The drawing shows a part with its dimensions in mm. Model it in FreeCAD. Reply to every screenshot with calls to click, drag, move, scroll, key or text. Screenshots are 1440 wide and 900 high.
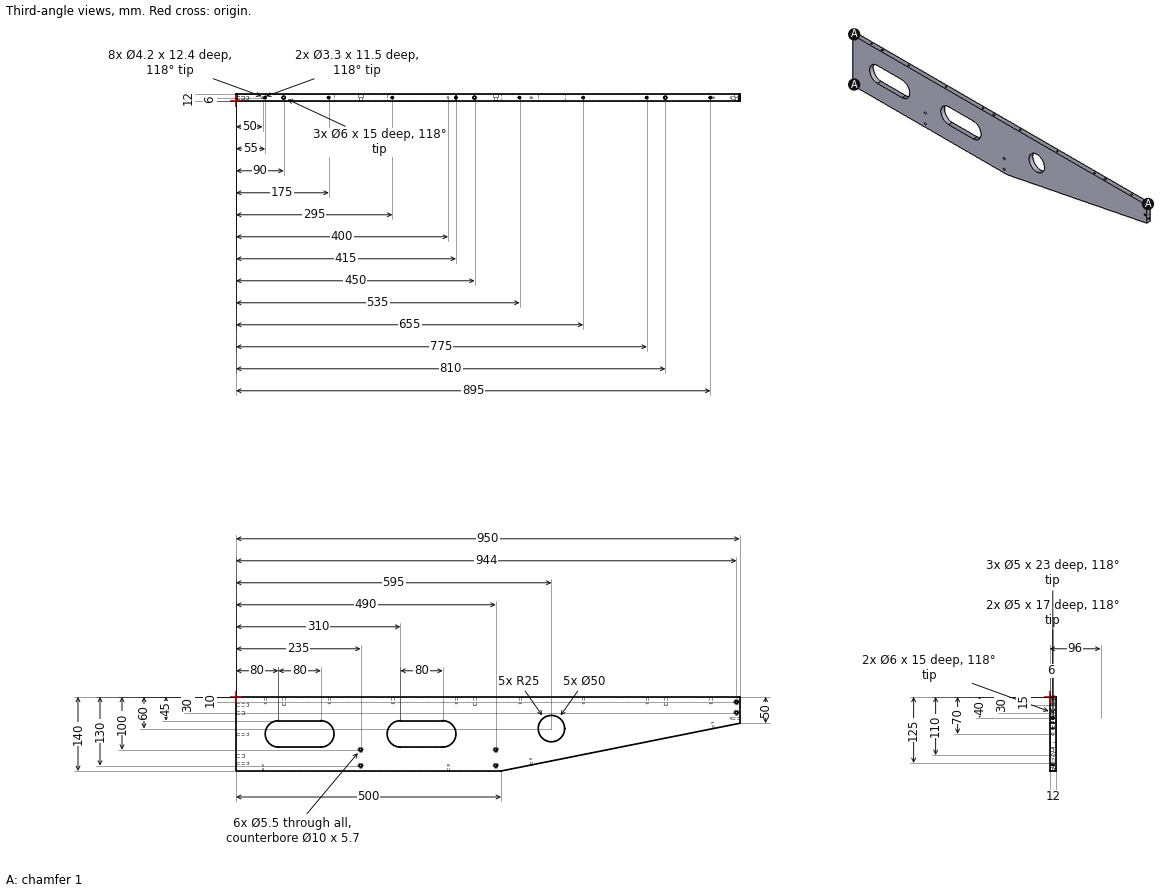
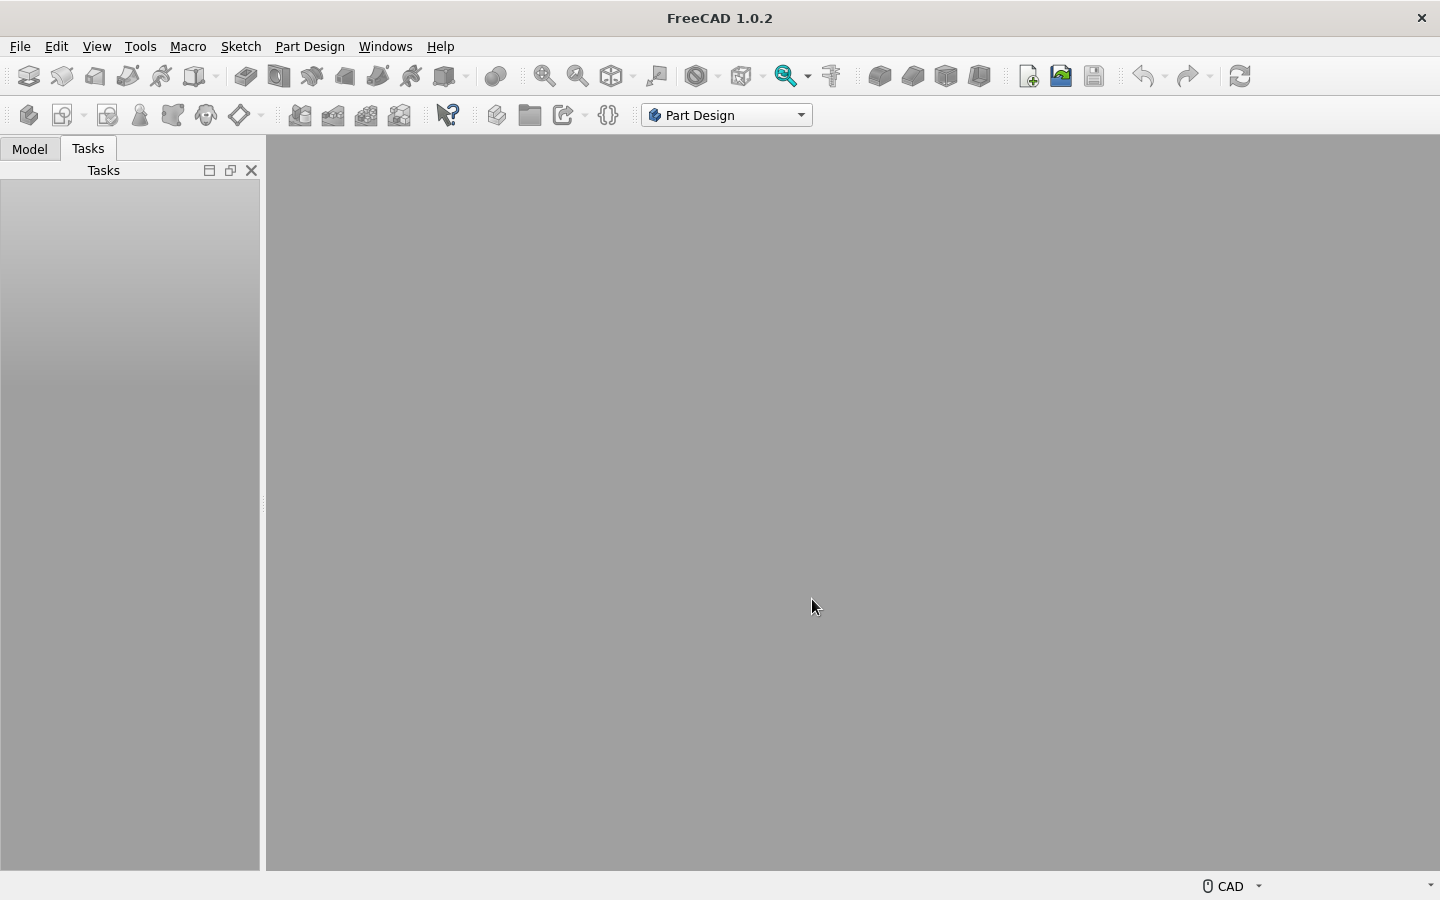
click(1028, 76)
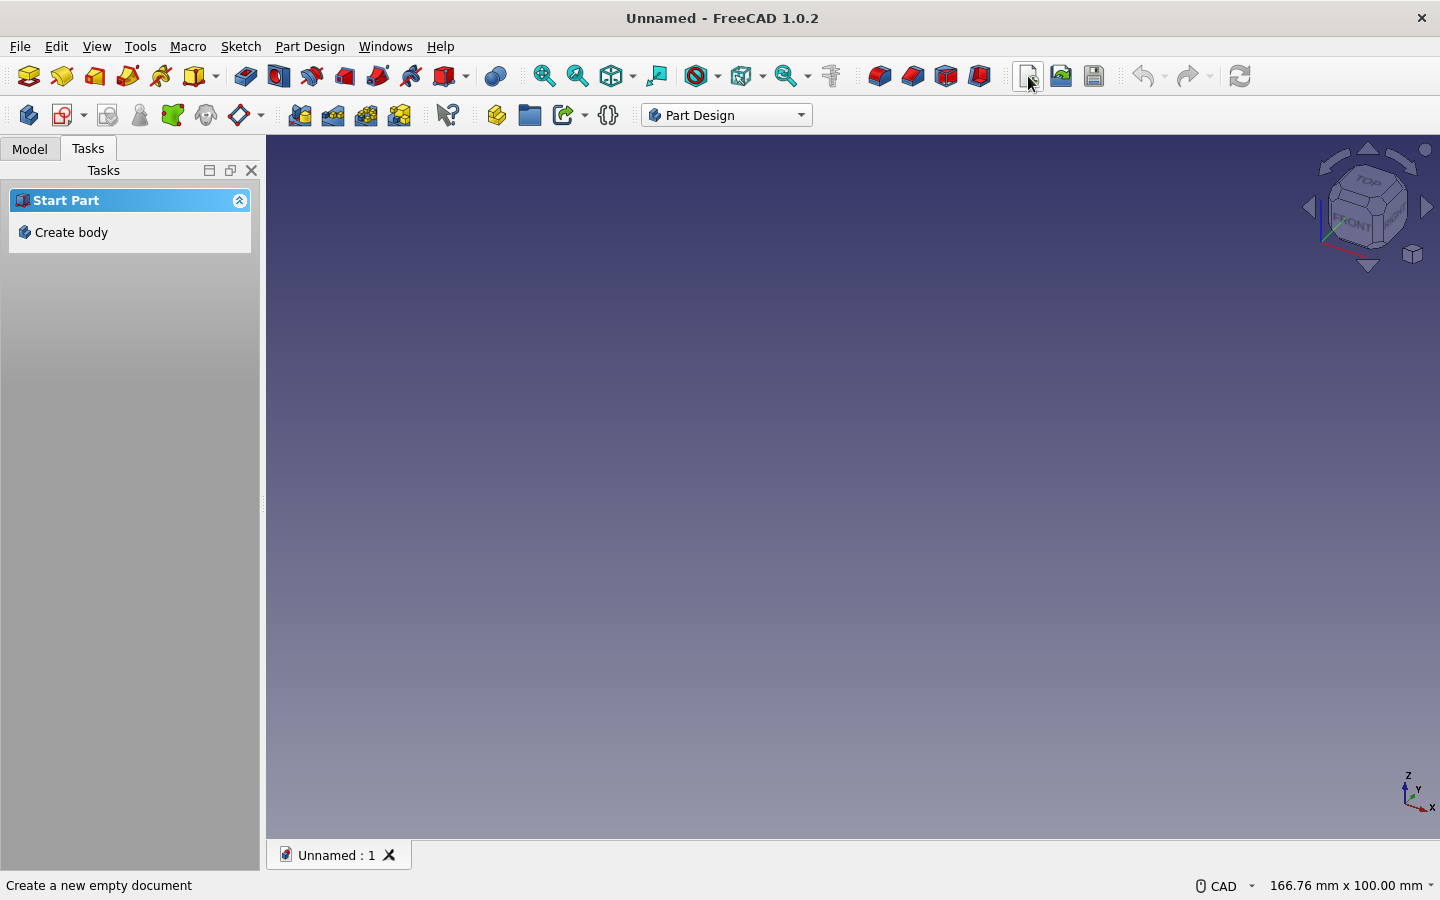
click(62, 116)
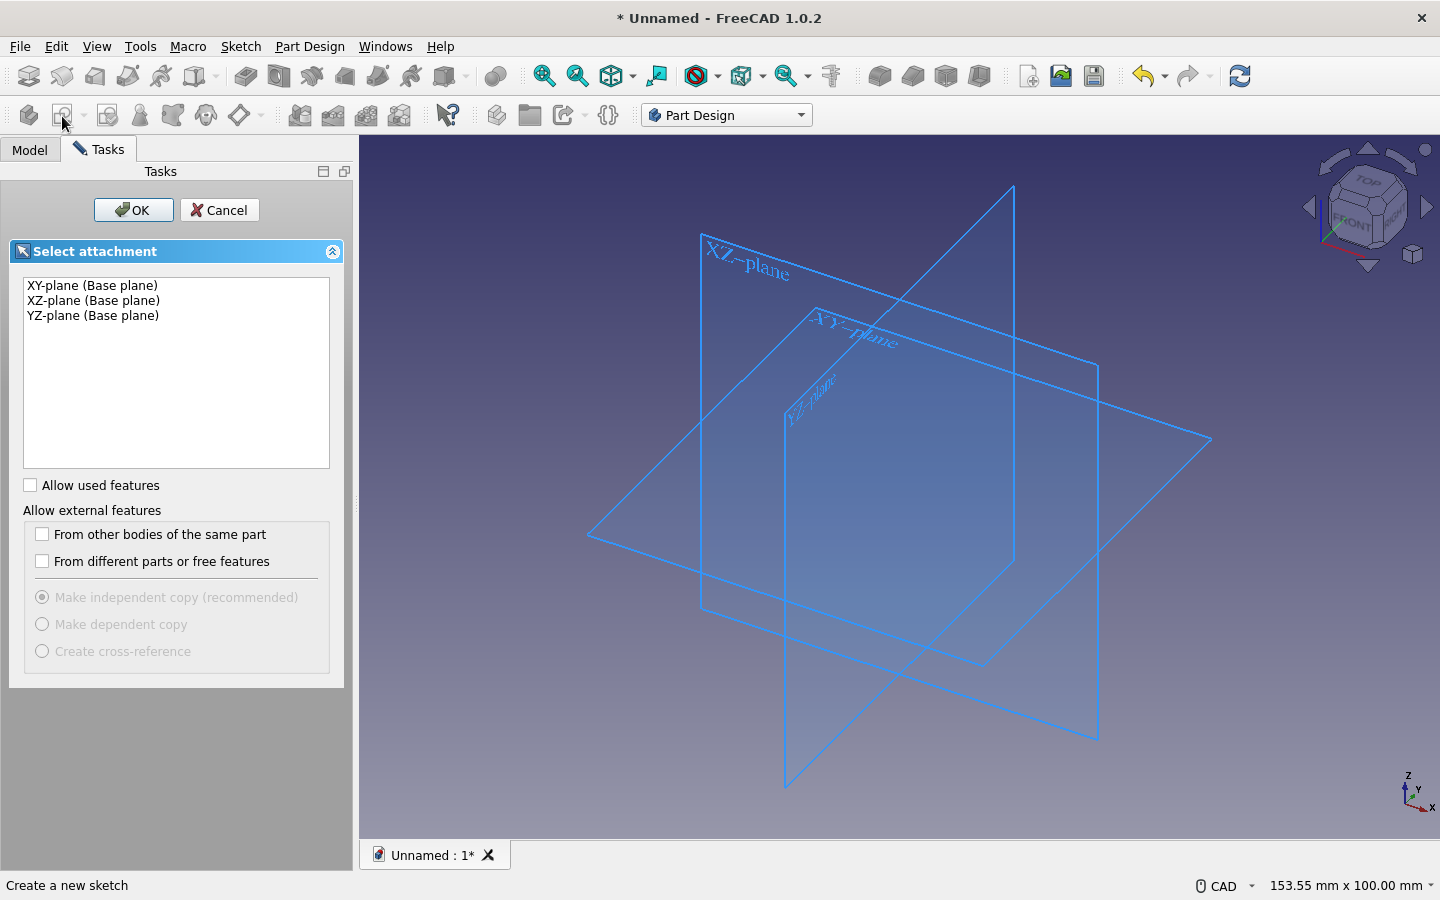
click(84, 300)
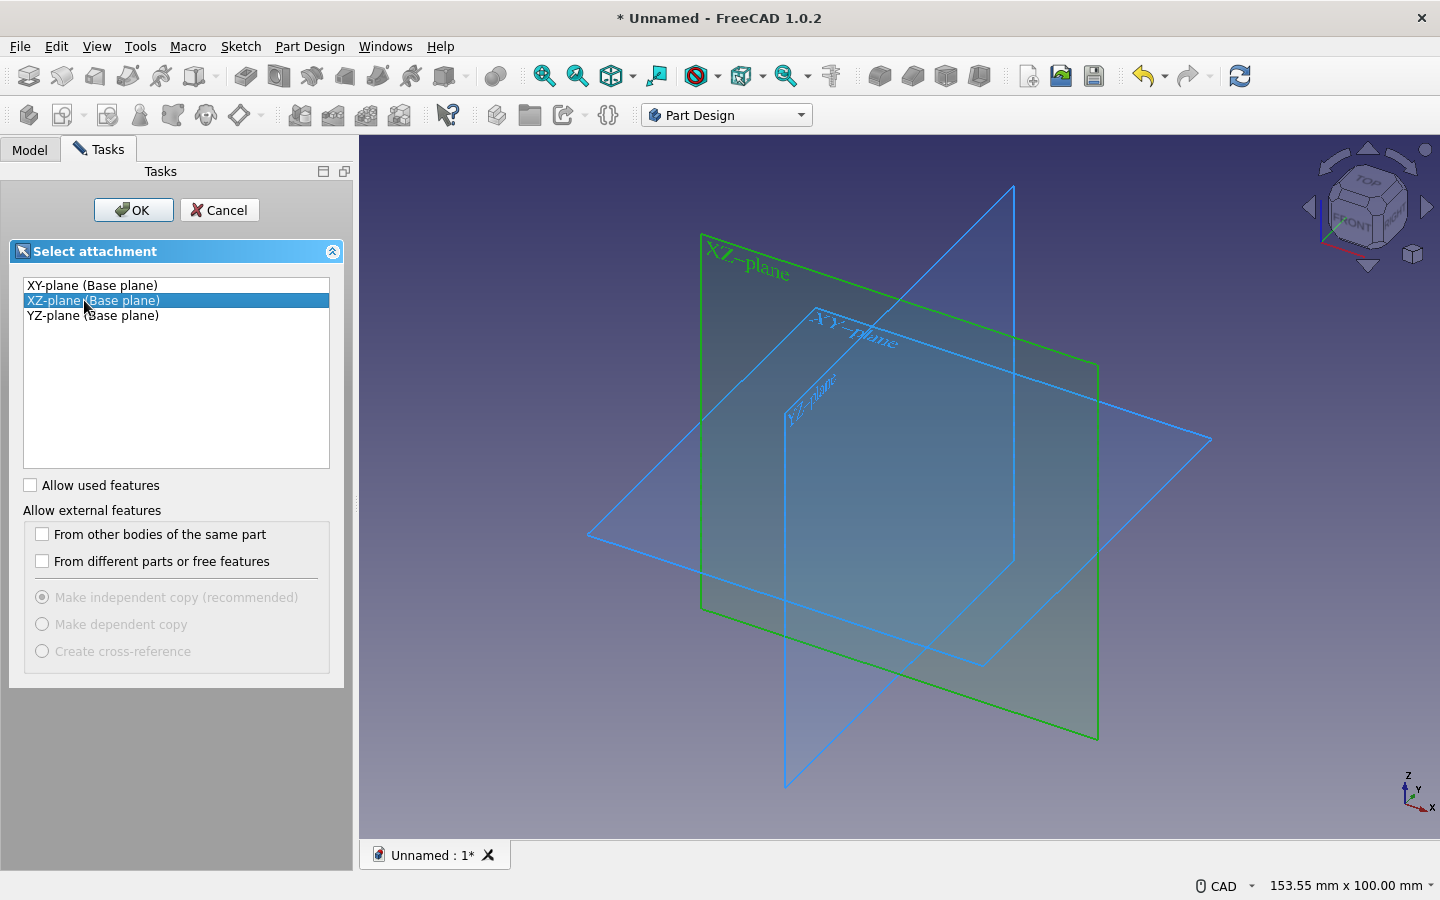
click(134, 210)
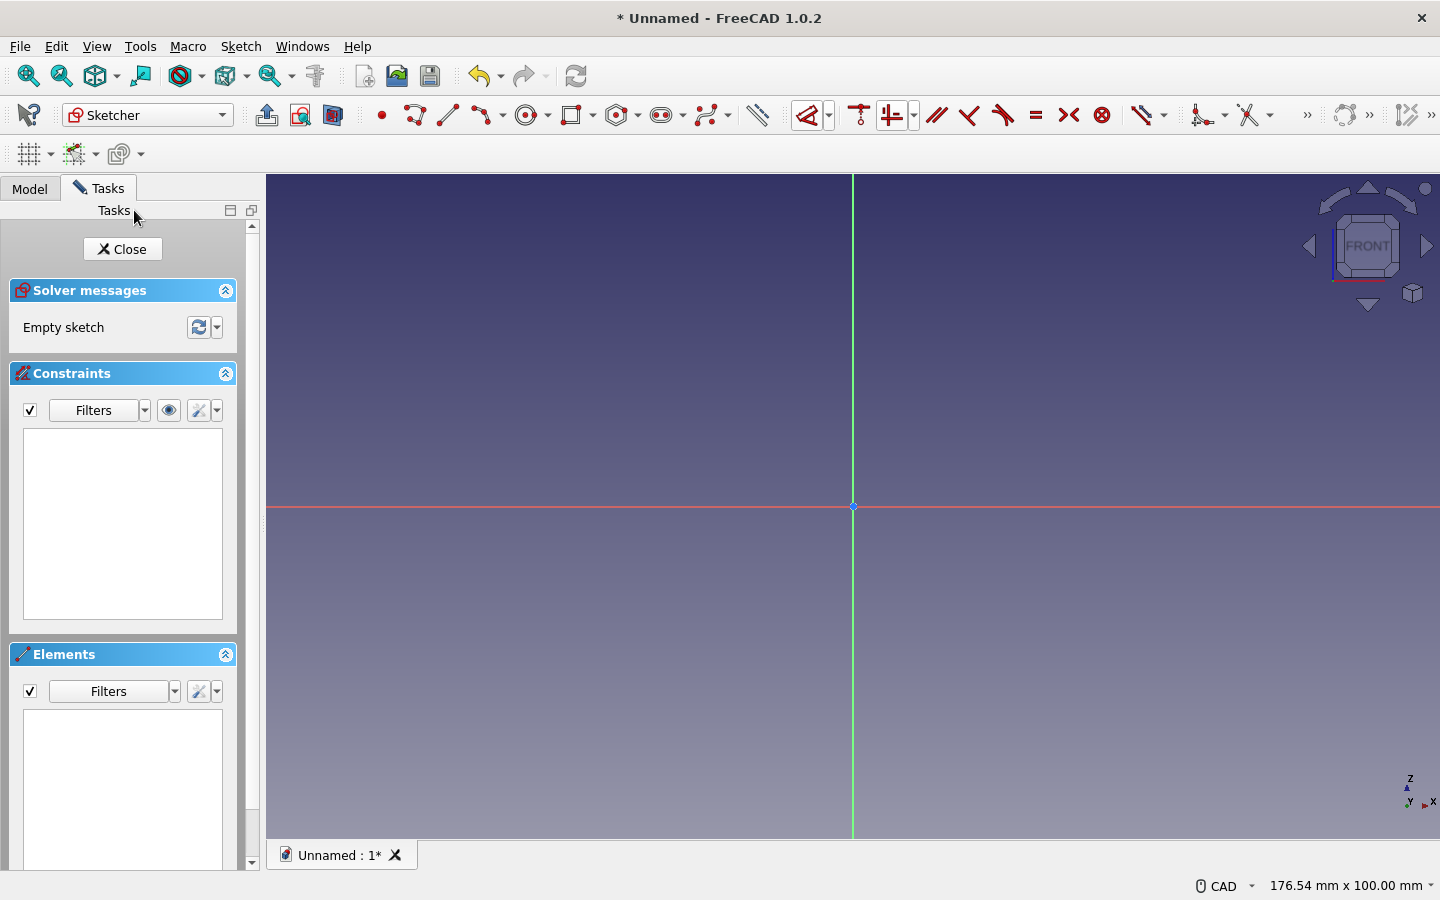
scroll(382, 448, down, 11)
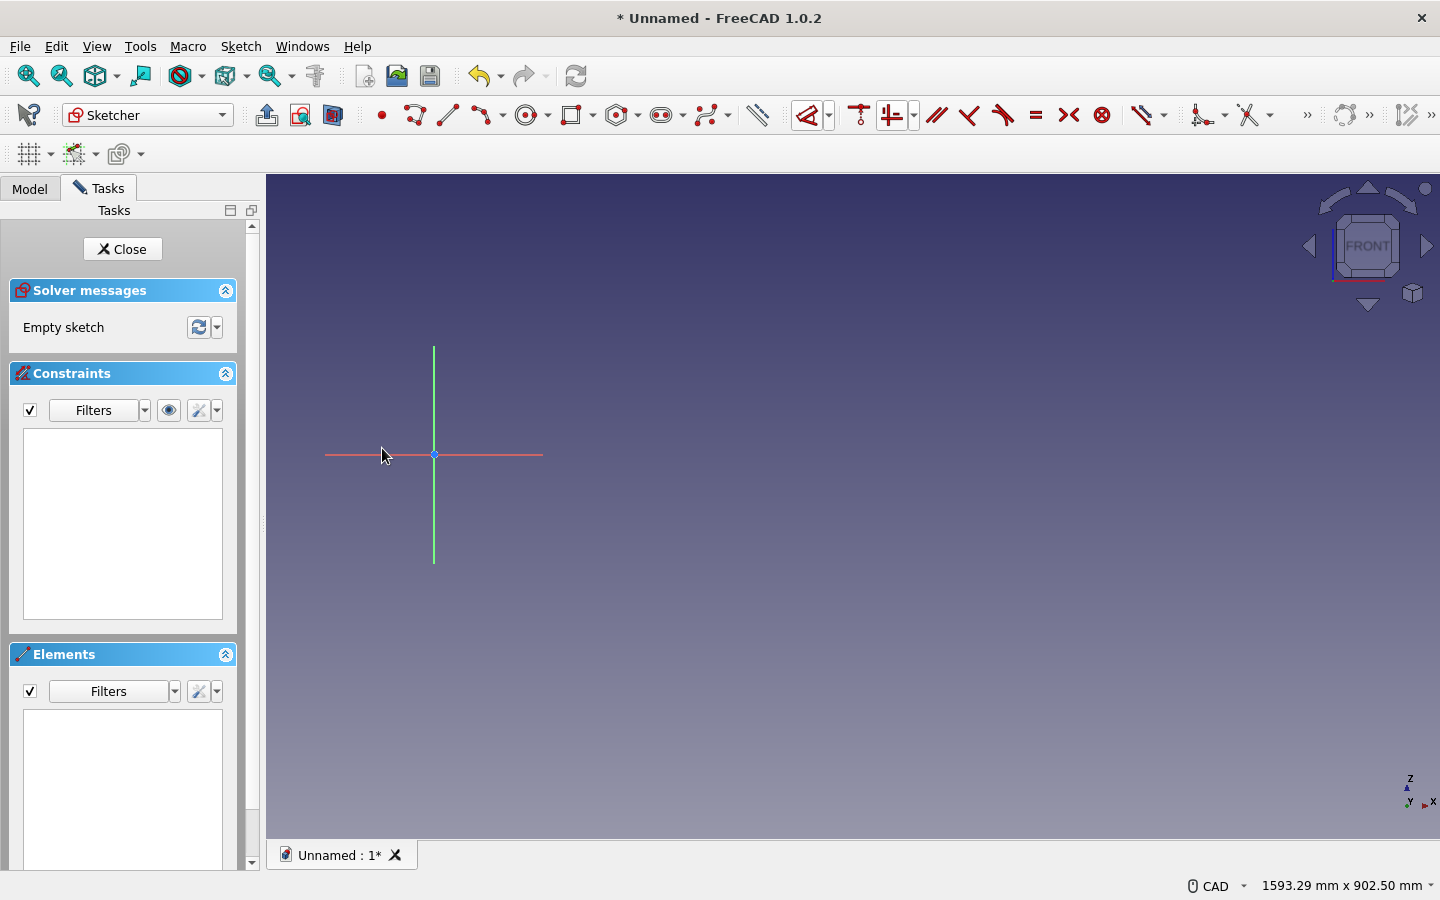
key(g)
key(m)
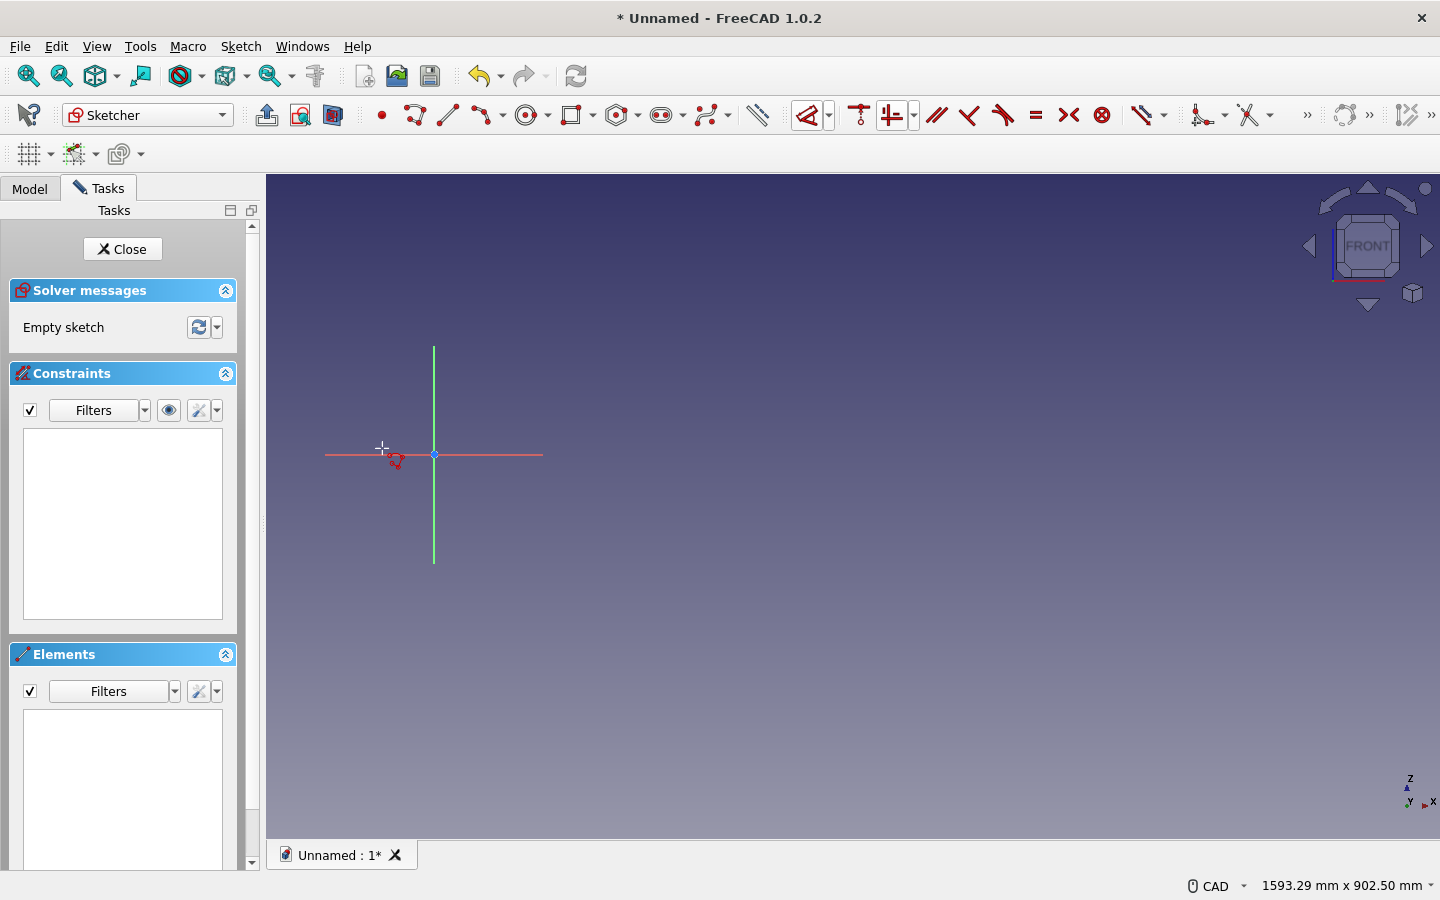
click(434, 455)
click(443, 558)
click(803, 558)
click(1134, 492)
click(1134, 464)
click(434, 455)
key(Escape)
key(Escape)